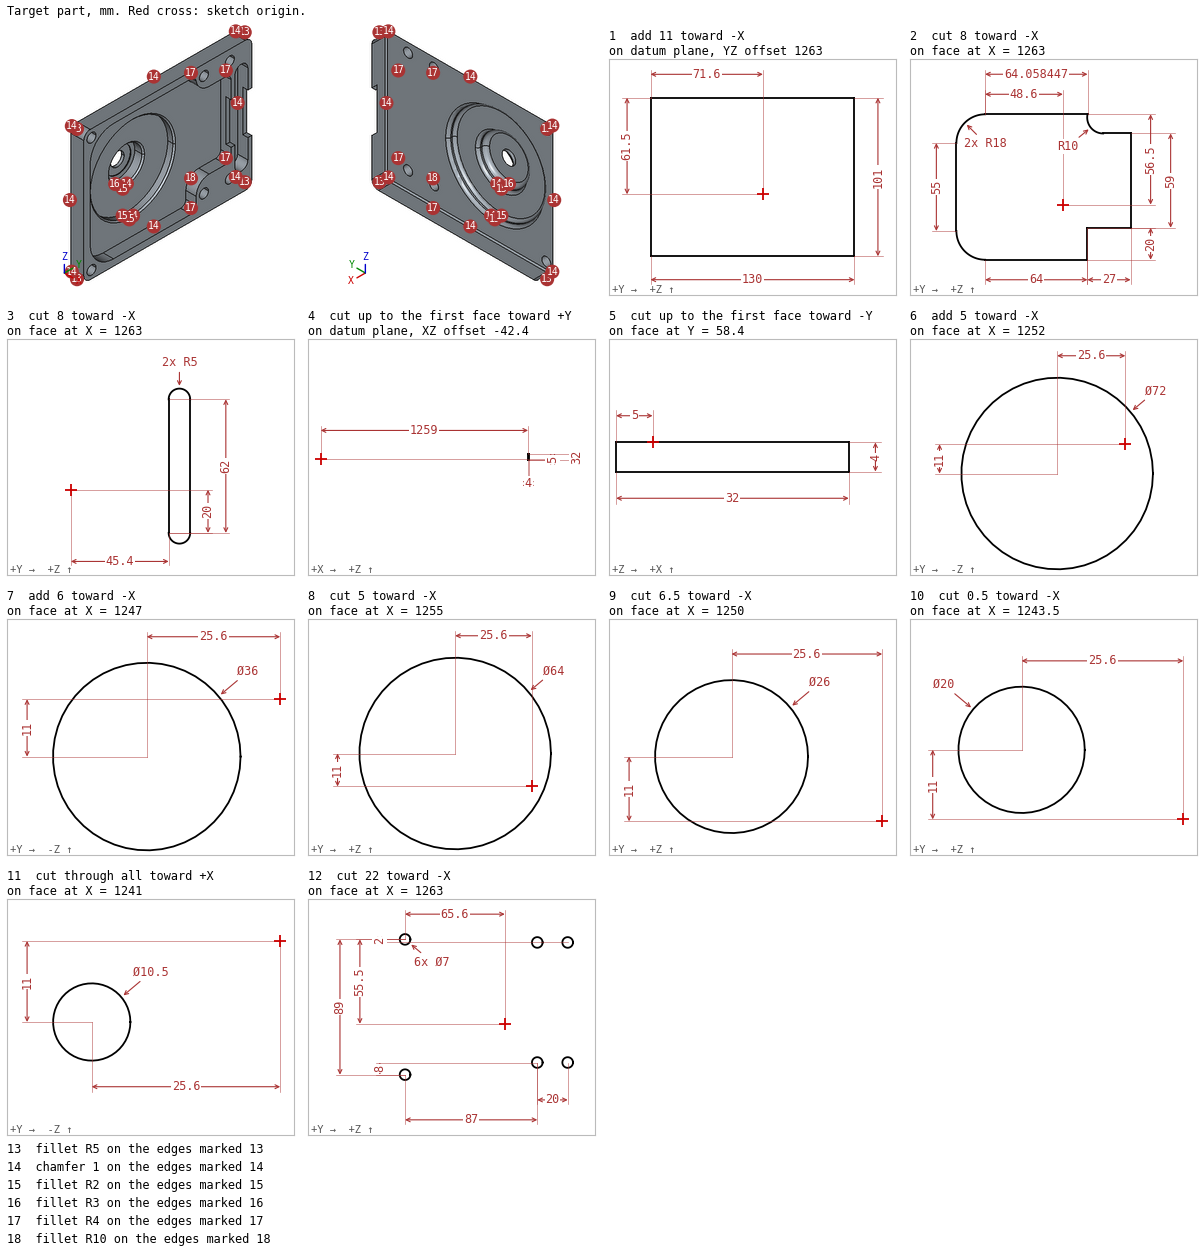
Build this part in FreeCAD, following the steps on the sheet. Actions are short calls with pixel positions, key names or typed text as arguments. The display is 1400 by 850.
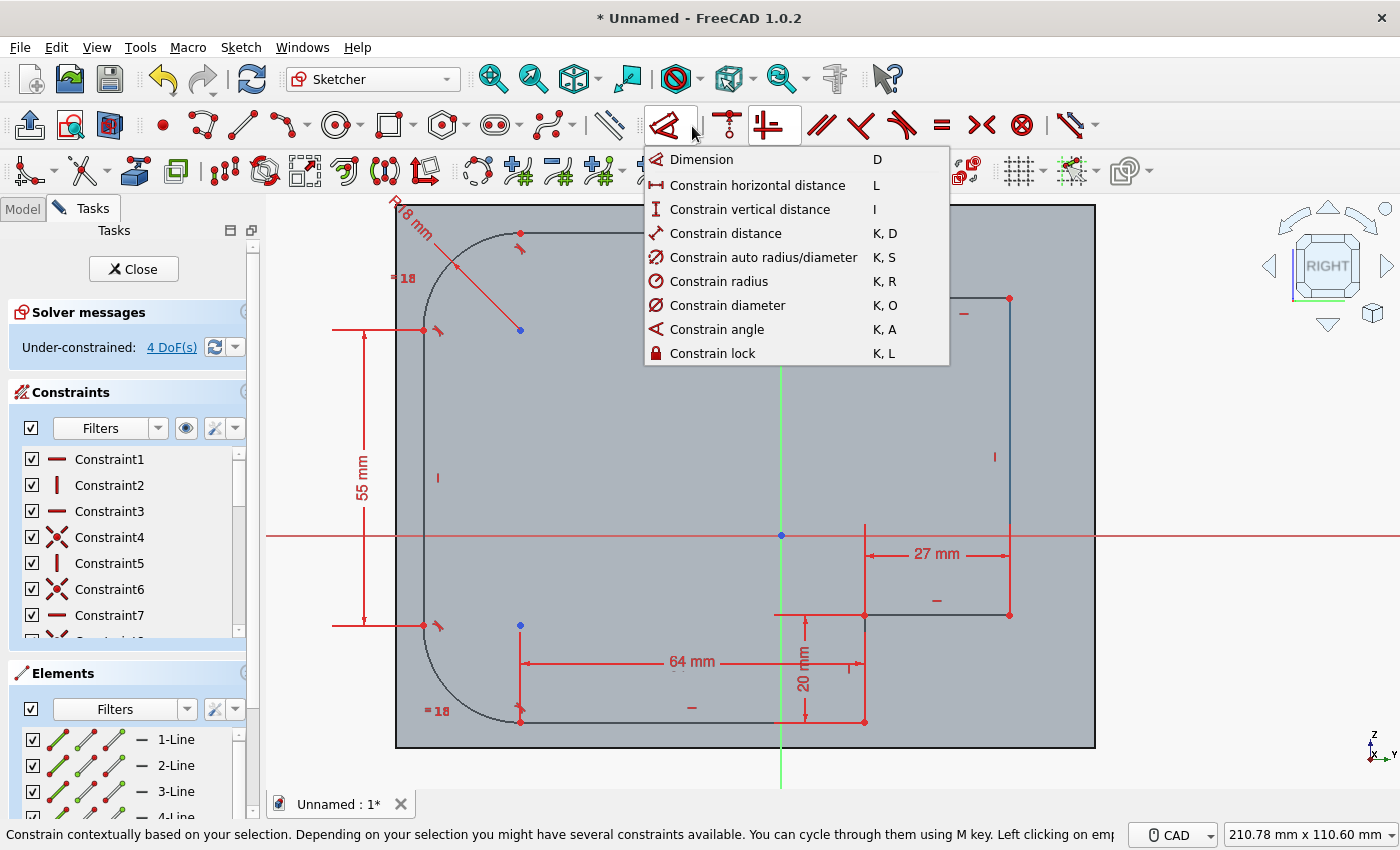
click(797, 209)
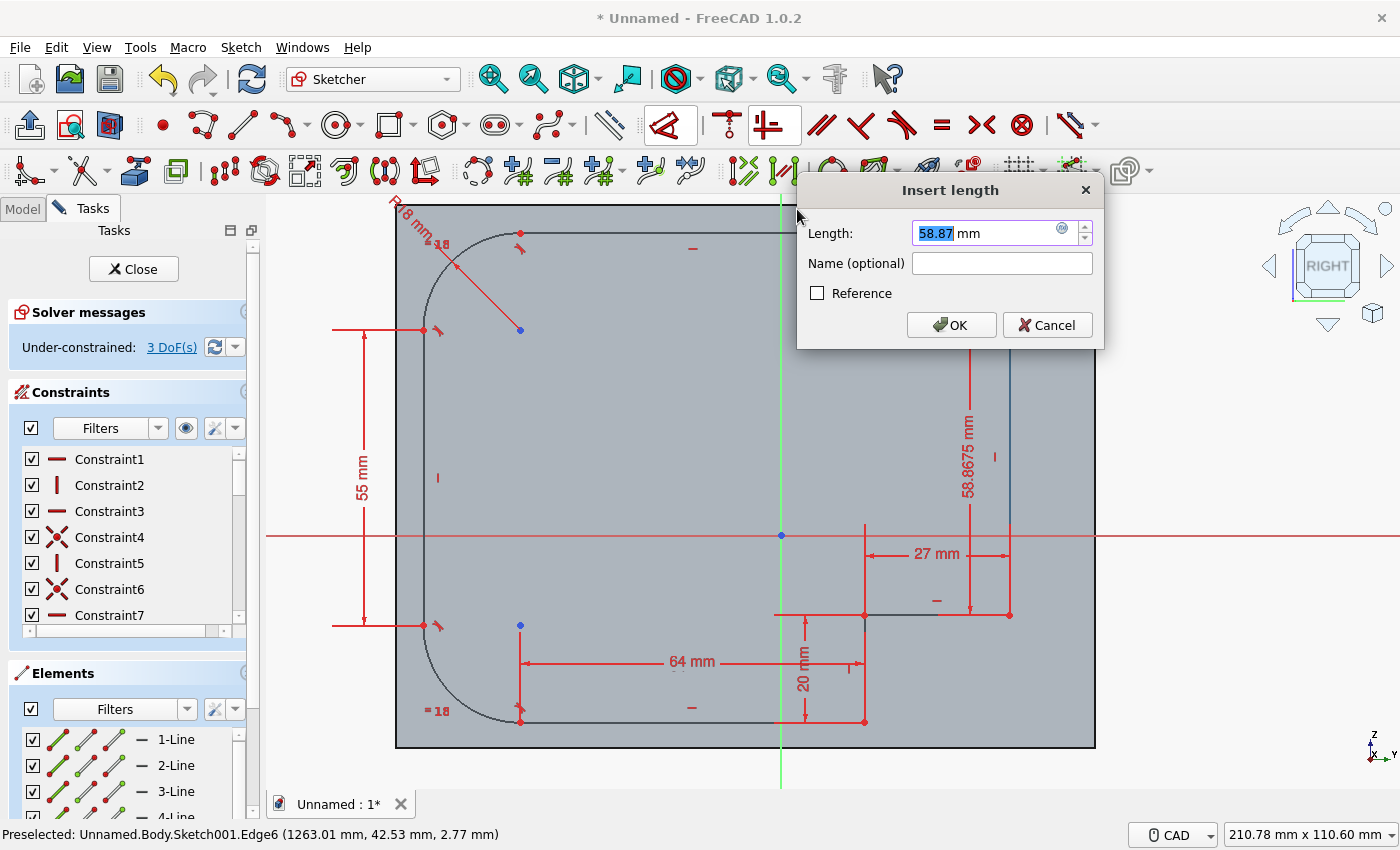
text(59)
key(Return)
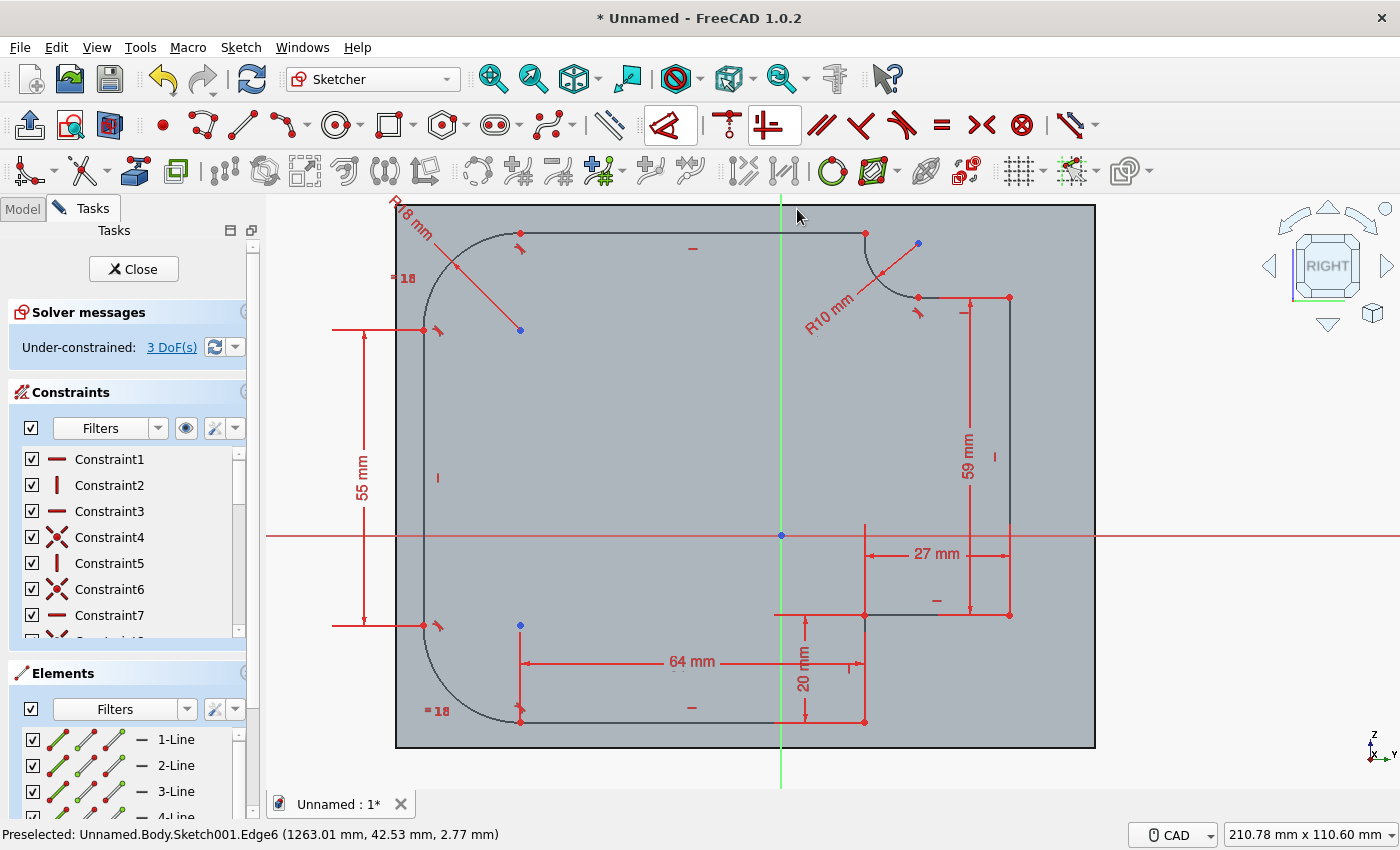
click(866, 233)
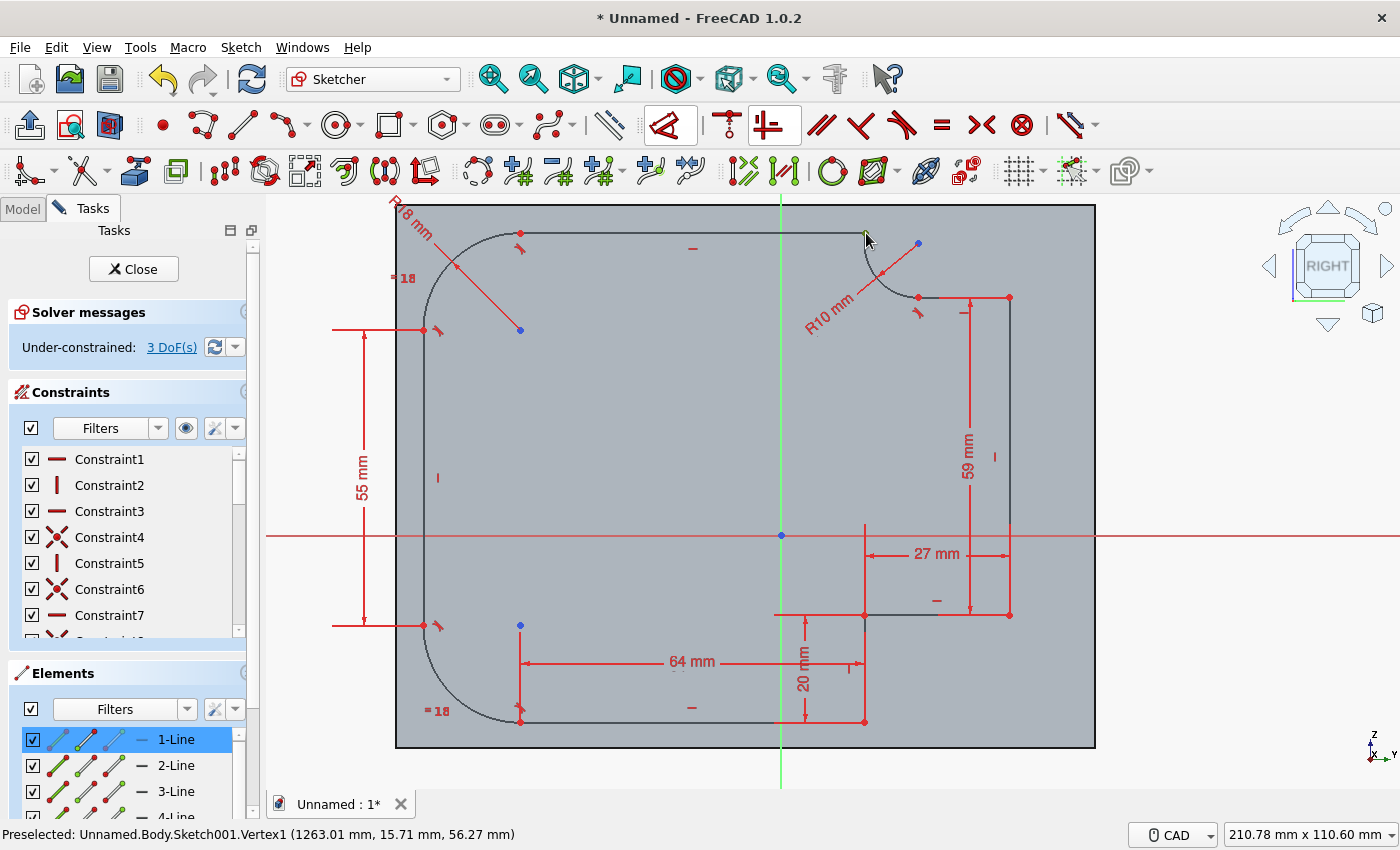
key(i)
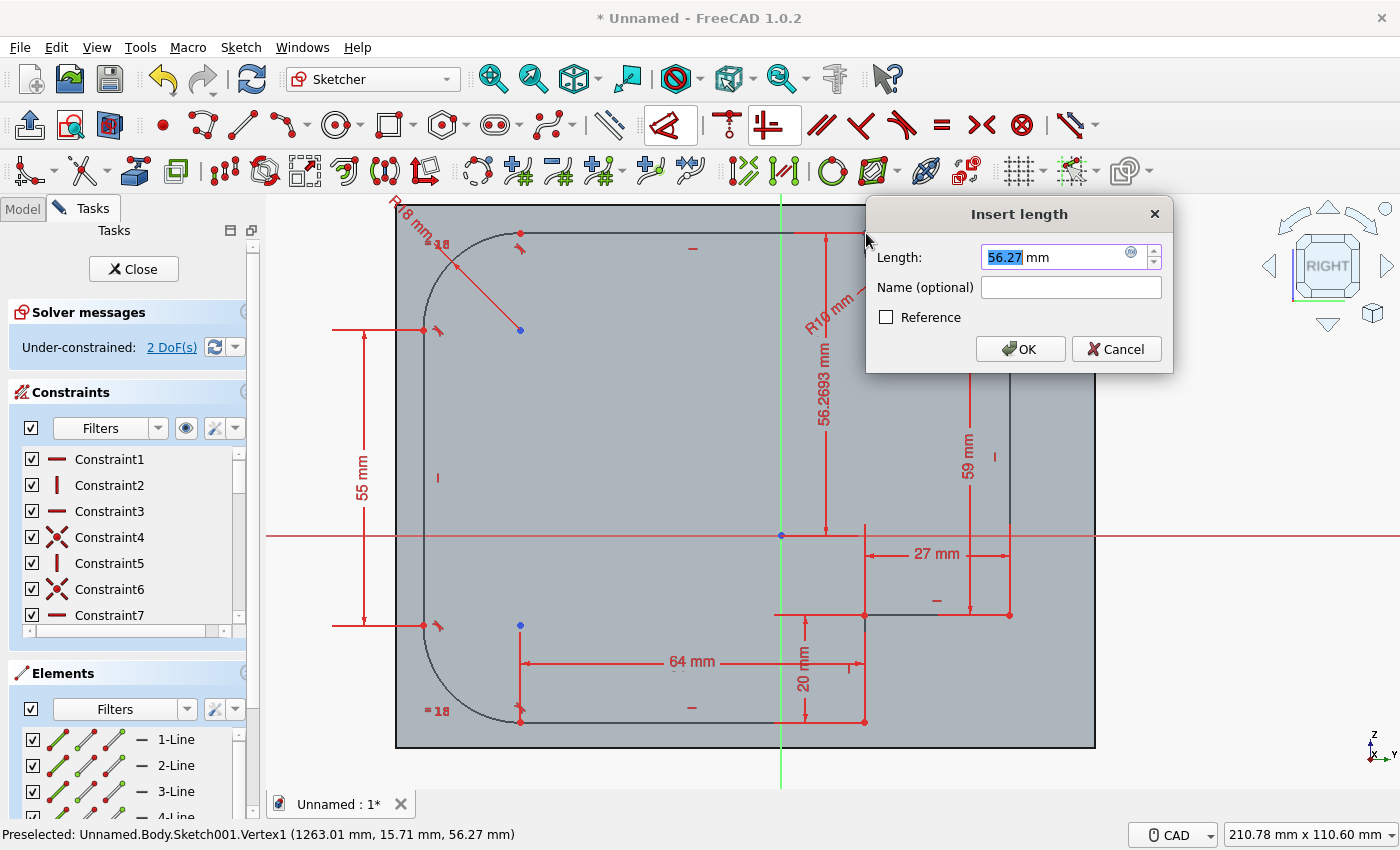
text(56.5)
key(Return)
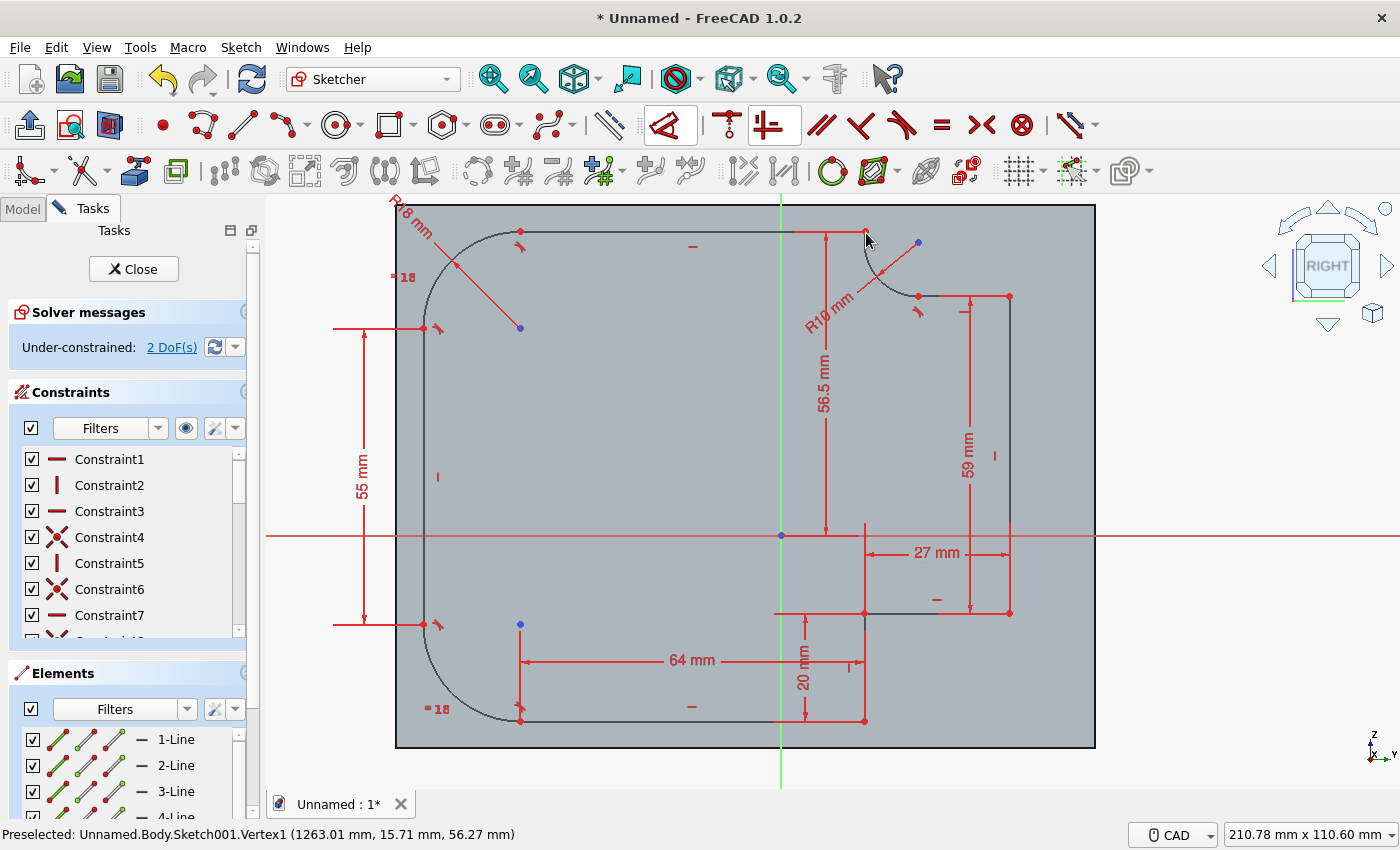
click(520, 232)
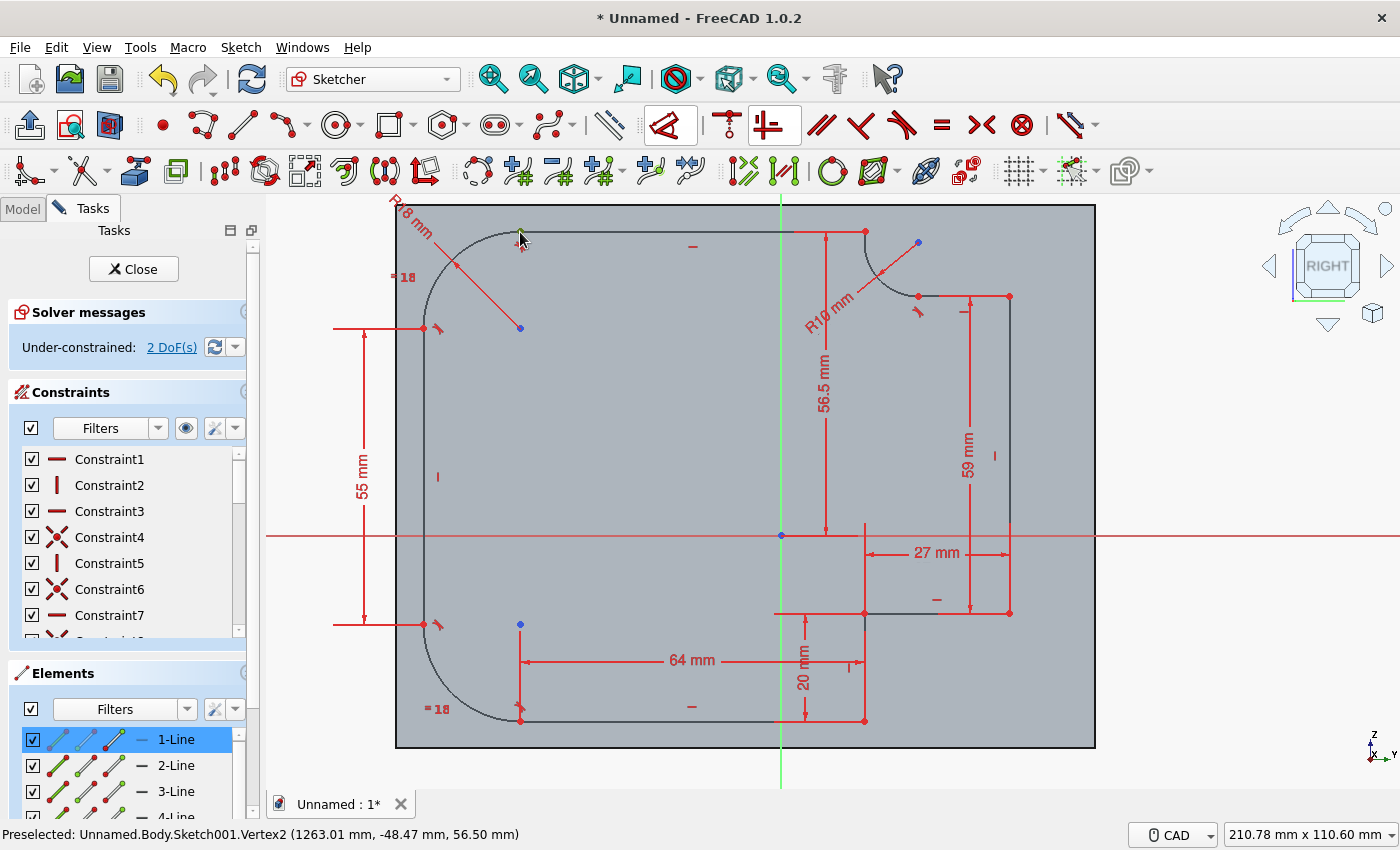
key(l)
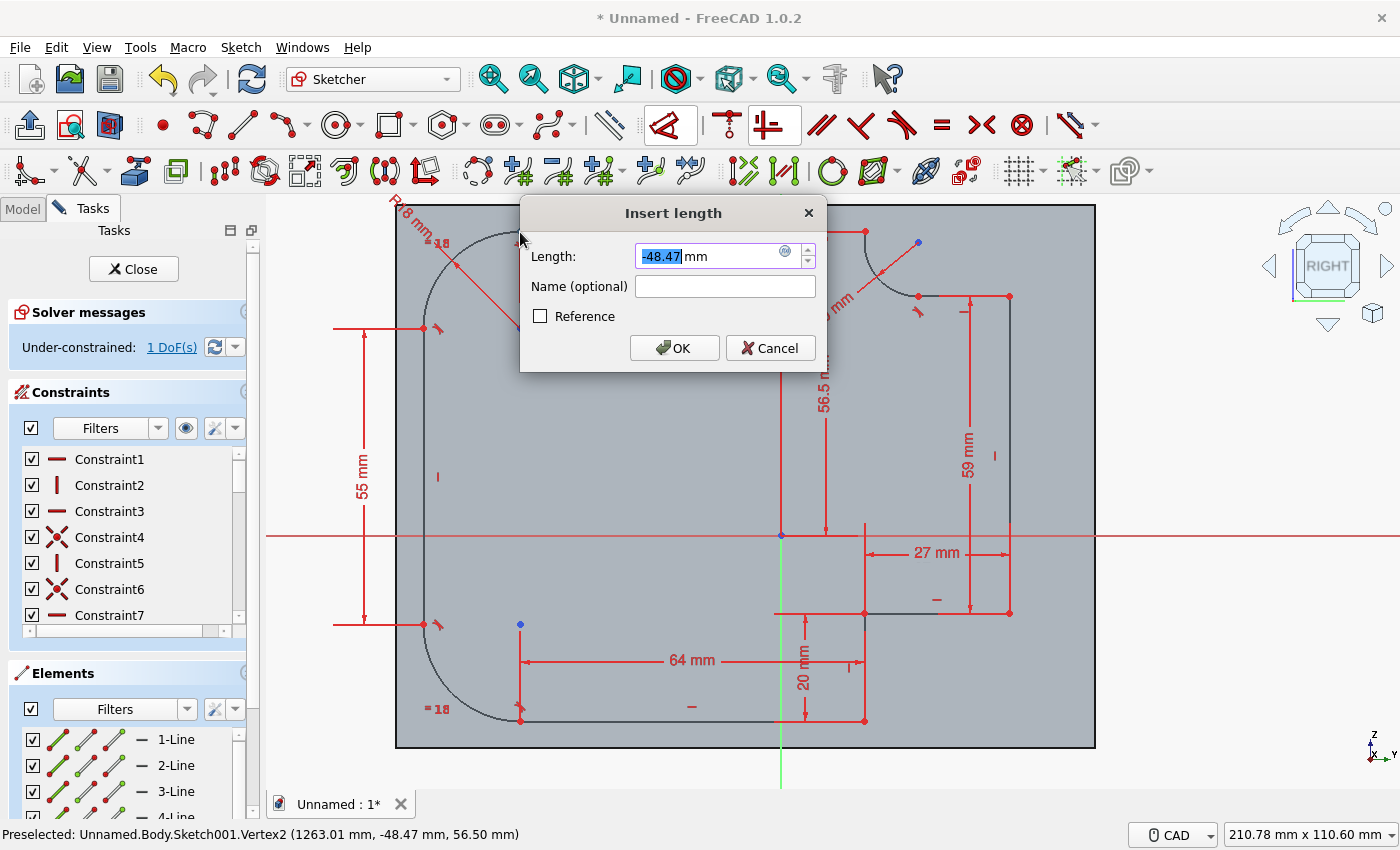
text(-48.6)
key(Return)